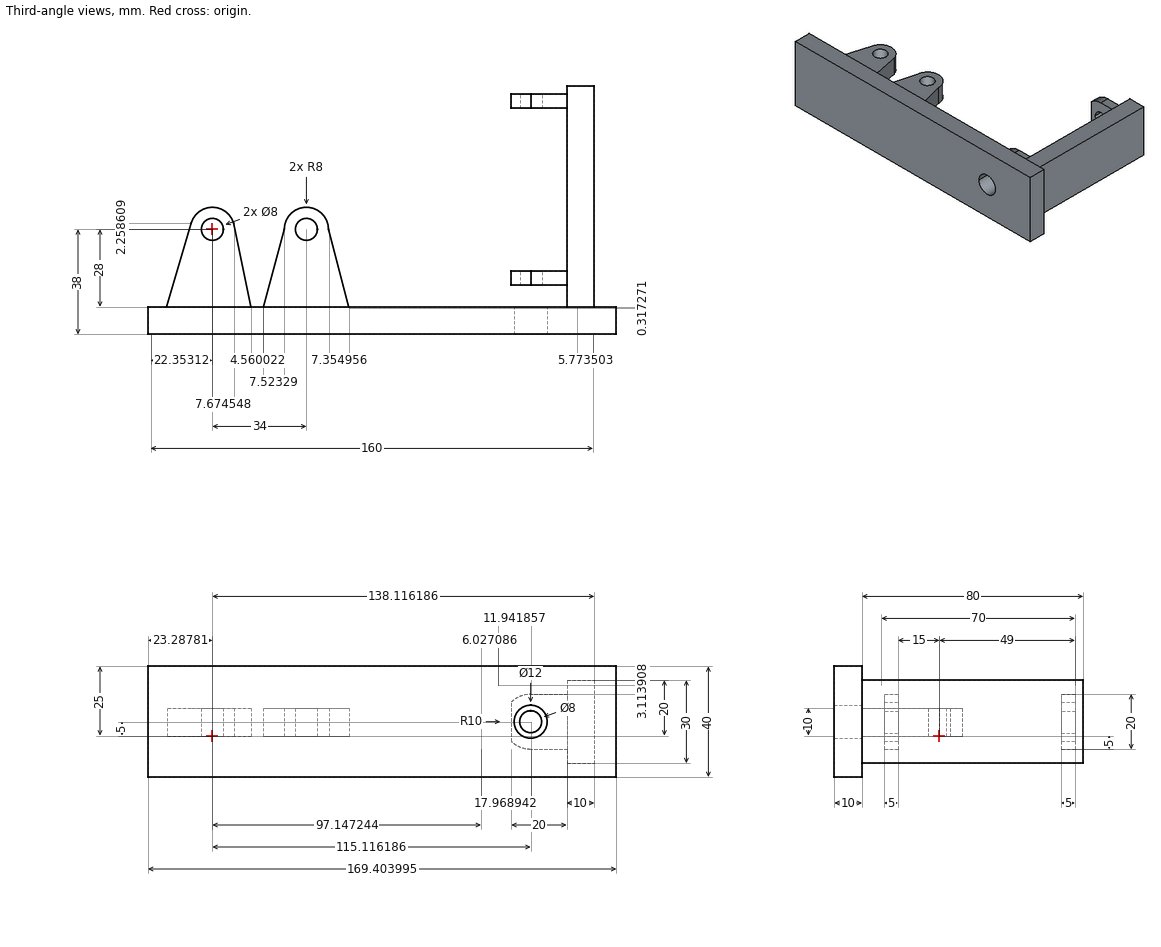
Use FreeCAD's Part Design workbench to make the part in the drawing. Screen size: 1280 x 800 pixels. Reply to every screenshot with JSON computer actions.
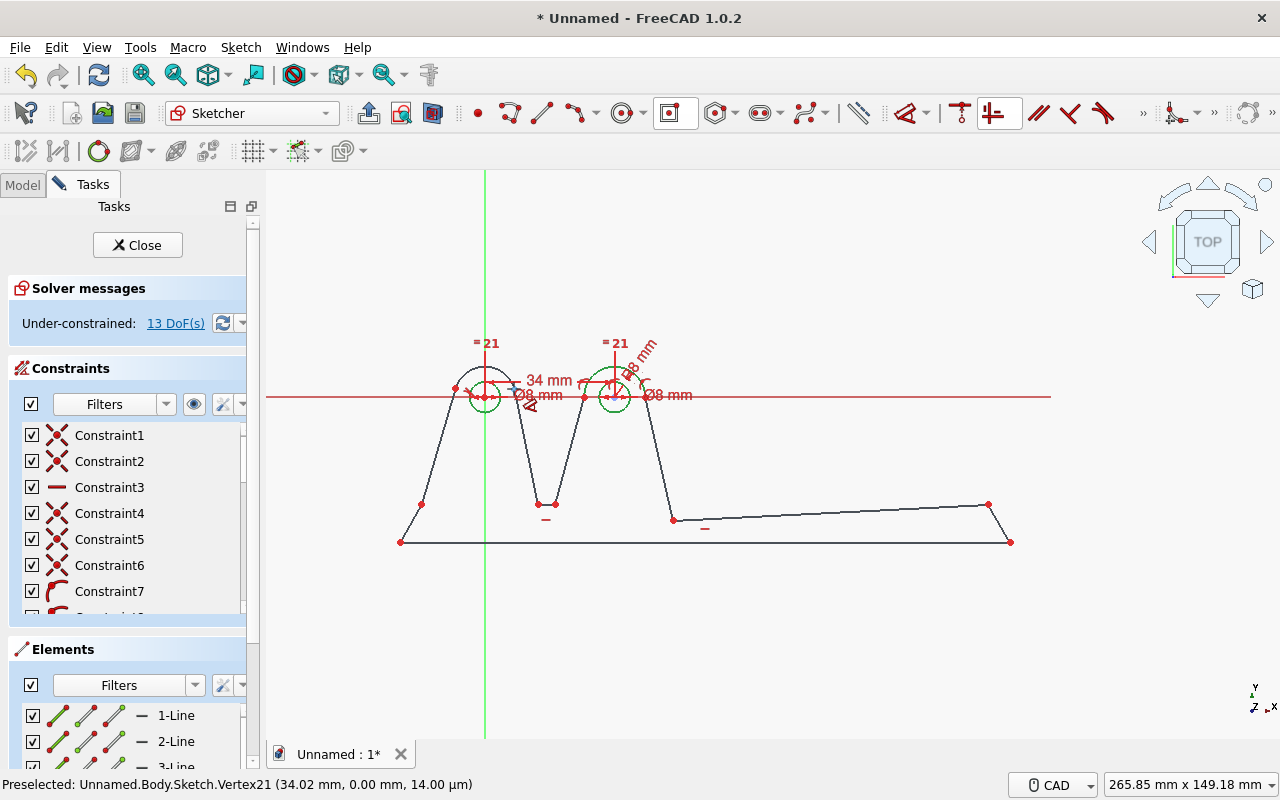
{"action": "left_click", "coordinate": [583, 543]}
{"action": "left_click", "coordinate": [705, 577]}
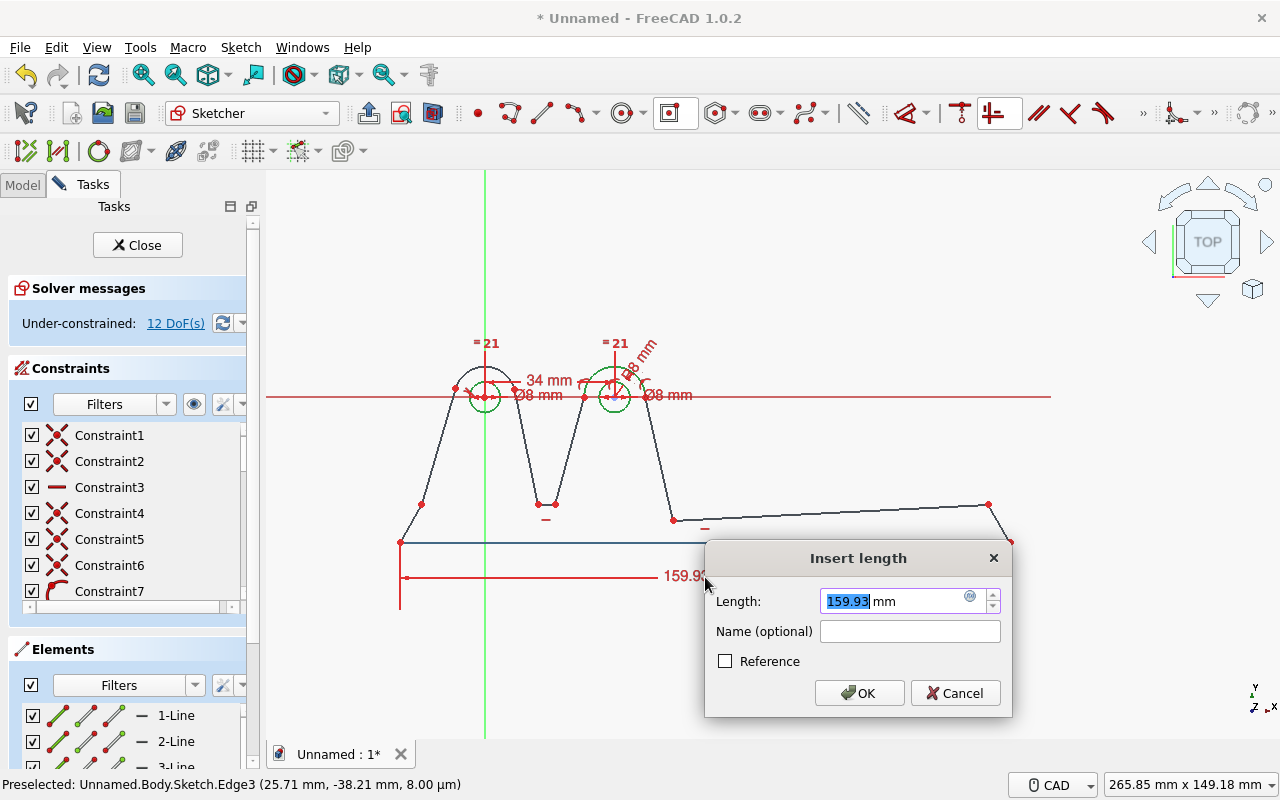
{"action": "type", "text": "160"}
{"action": "key", "text": "Return"}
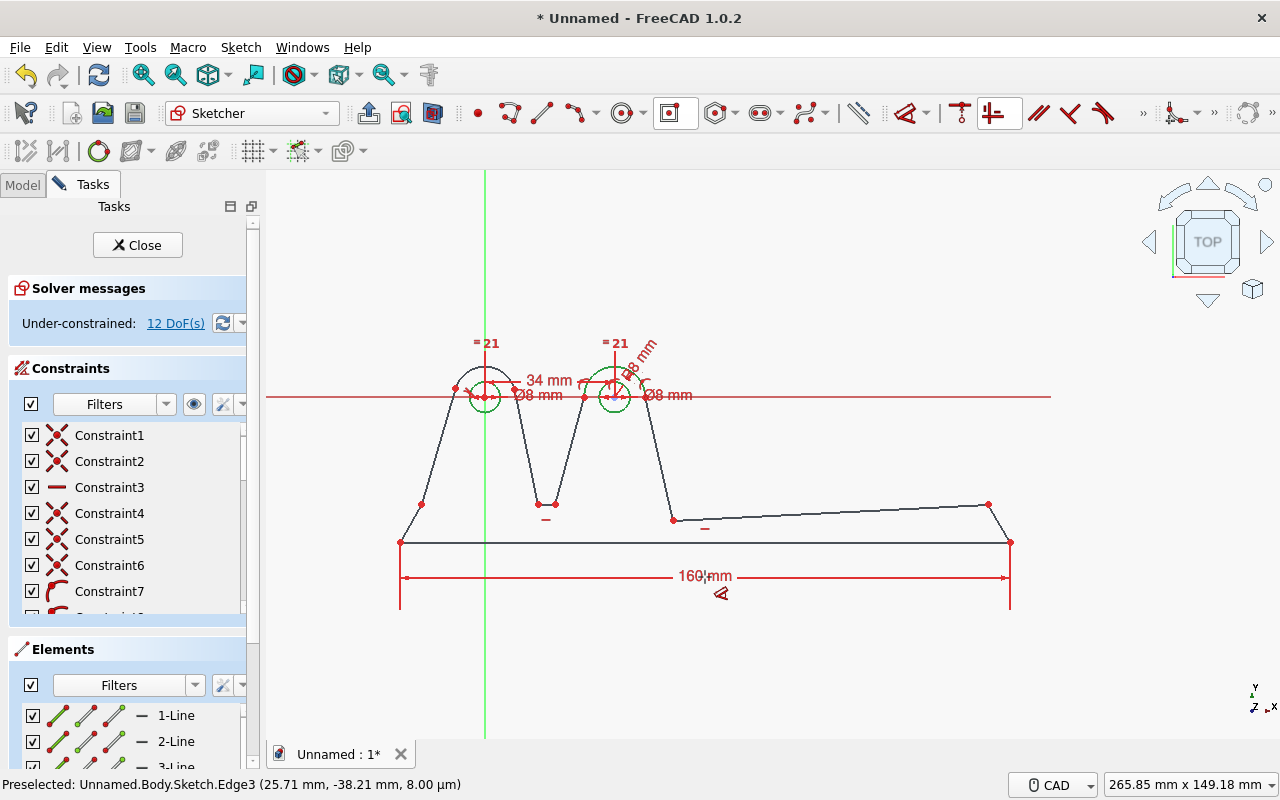
{"action": "left_click", "coordinate": [422, 505]}
{"action": "left_click", "coordinate": [388, 451]}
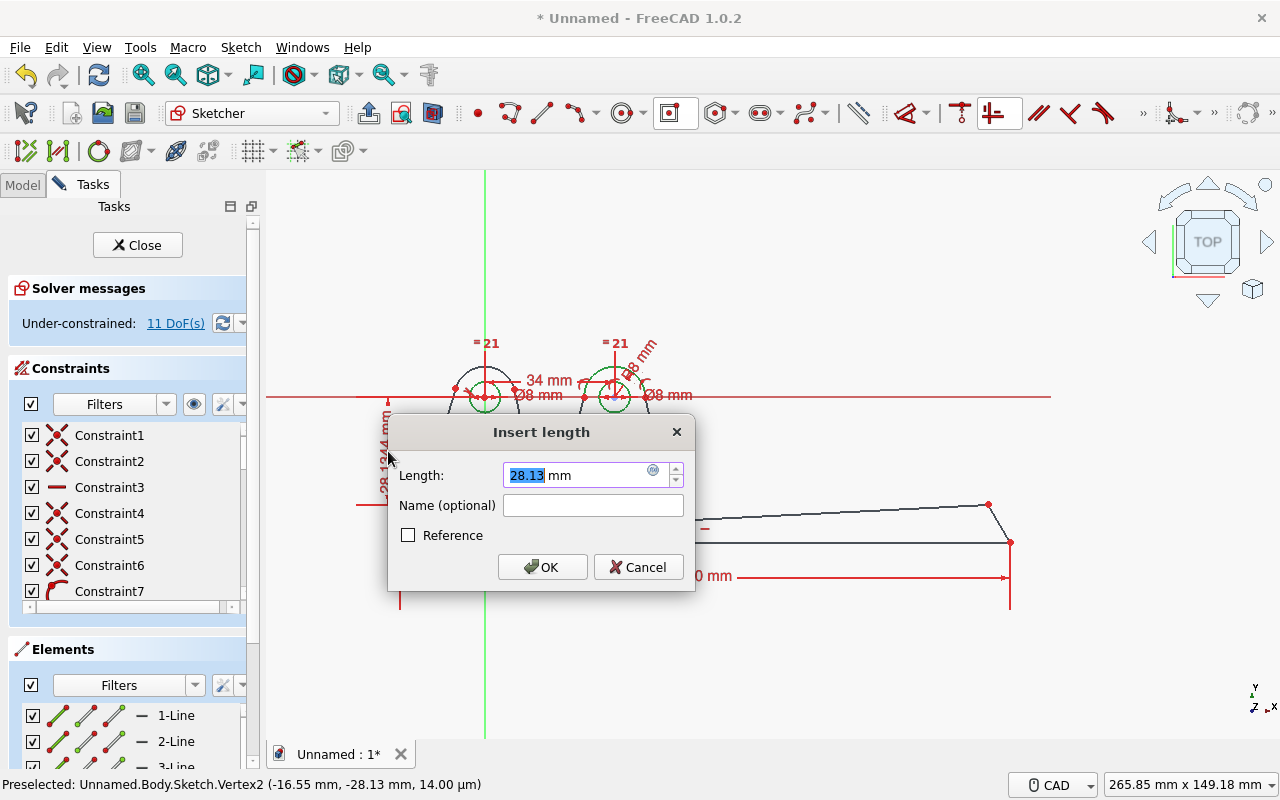
{"action": "type", "text": "28"}
{"action": "key", "text": "Return"}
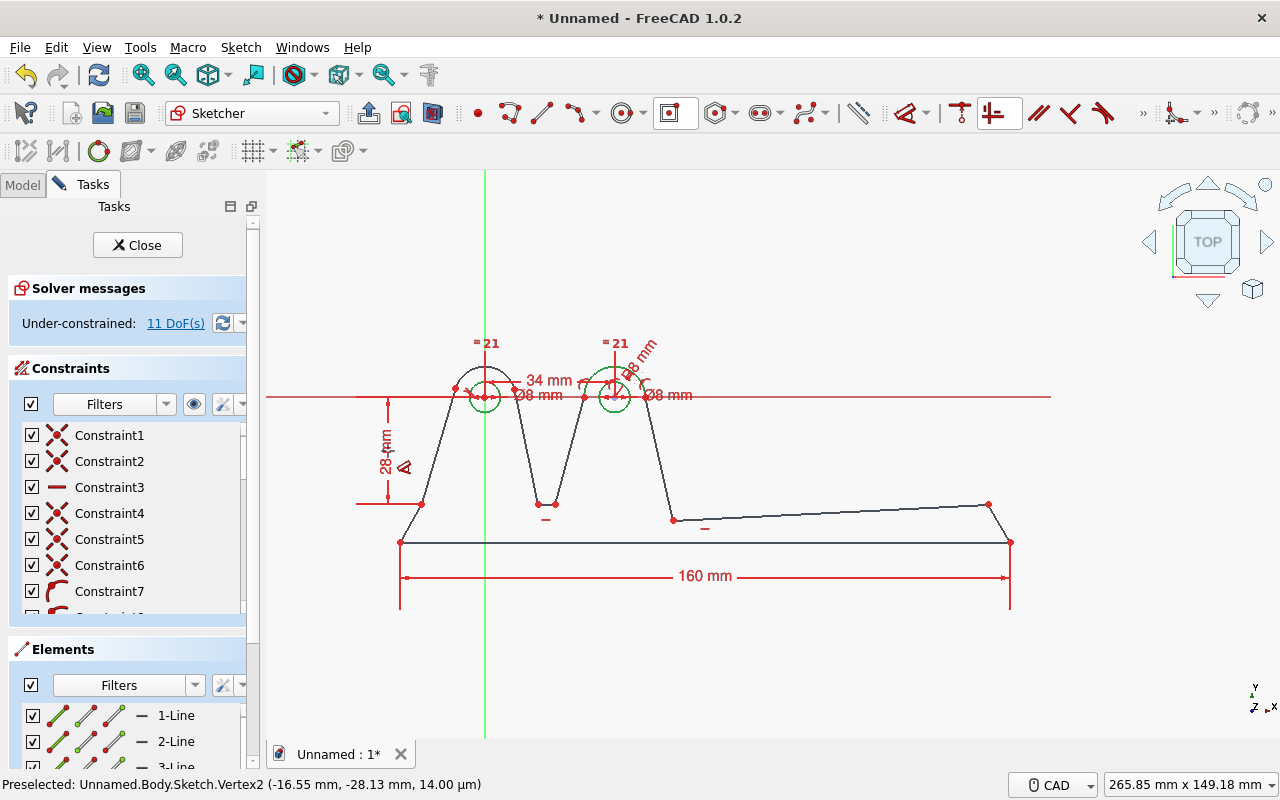
{"action": "left_click", "coordinate": [400, 543]}
{"action": "left_click", "coordinate": [366, 504]}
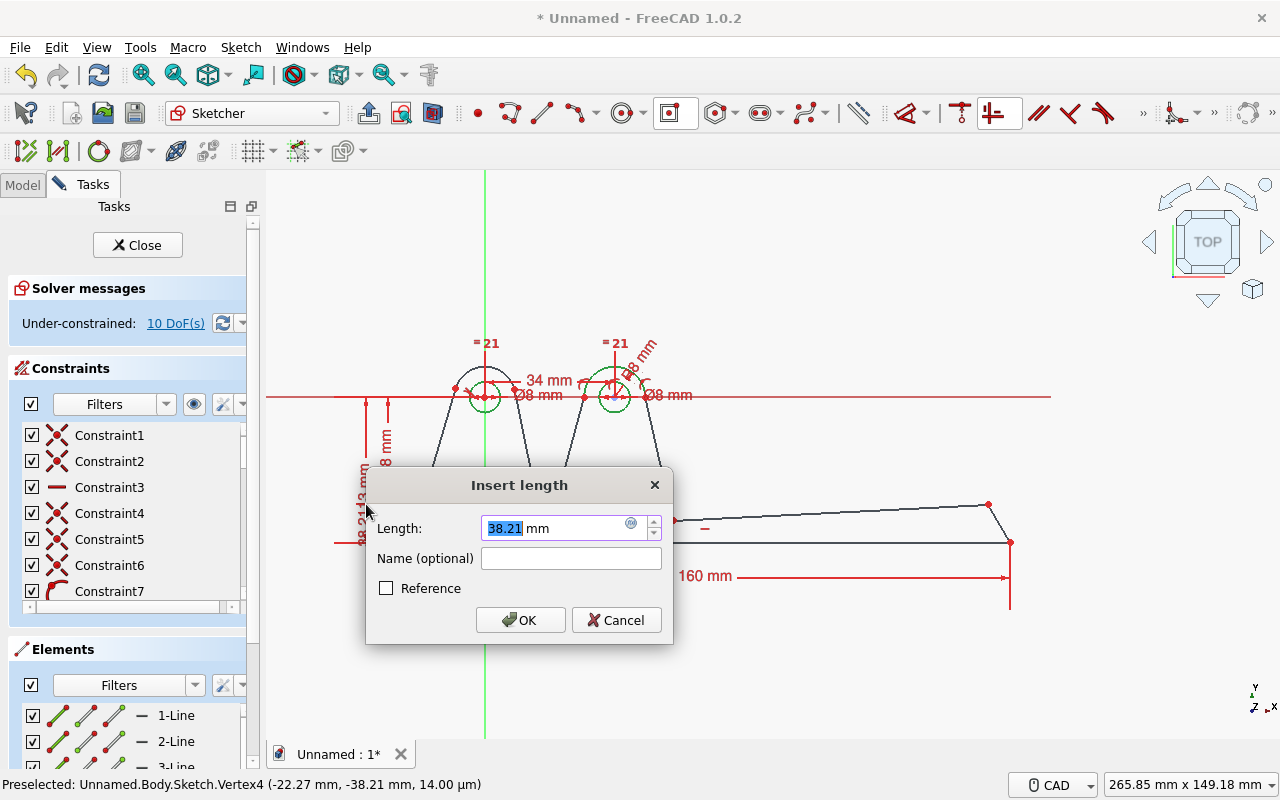
{"action": "type", "text": "38"}
{"action": "key", "text": "Return"}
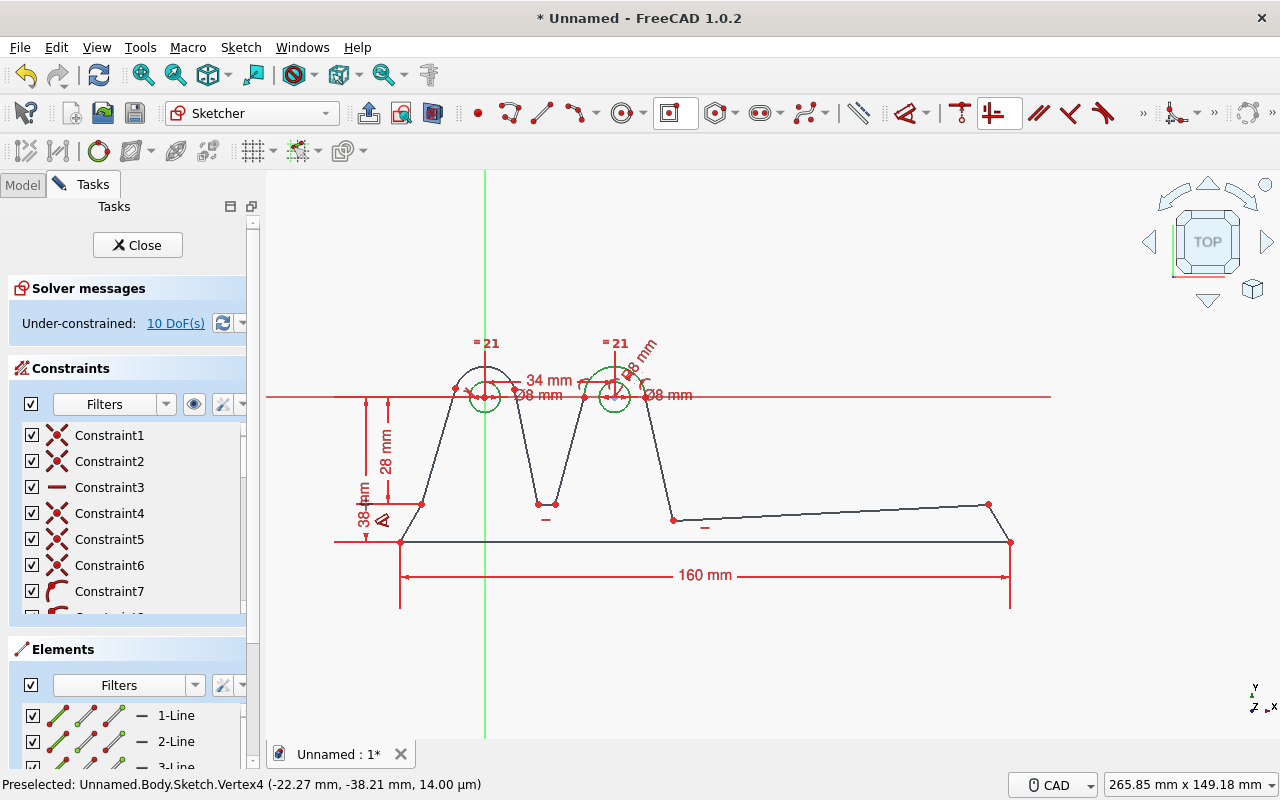
{"action": "left_click", "coordinate": [988, 505]}
{"action": "left_click", "coordinate": [1022, 451]}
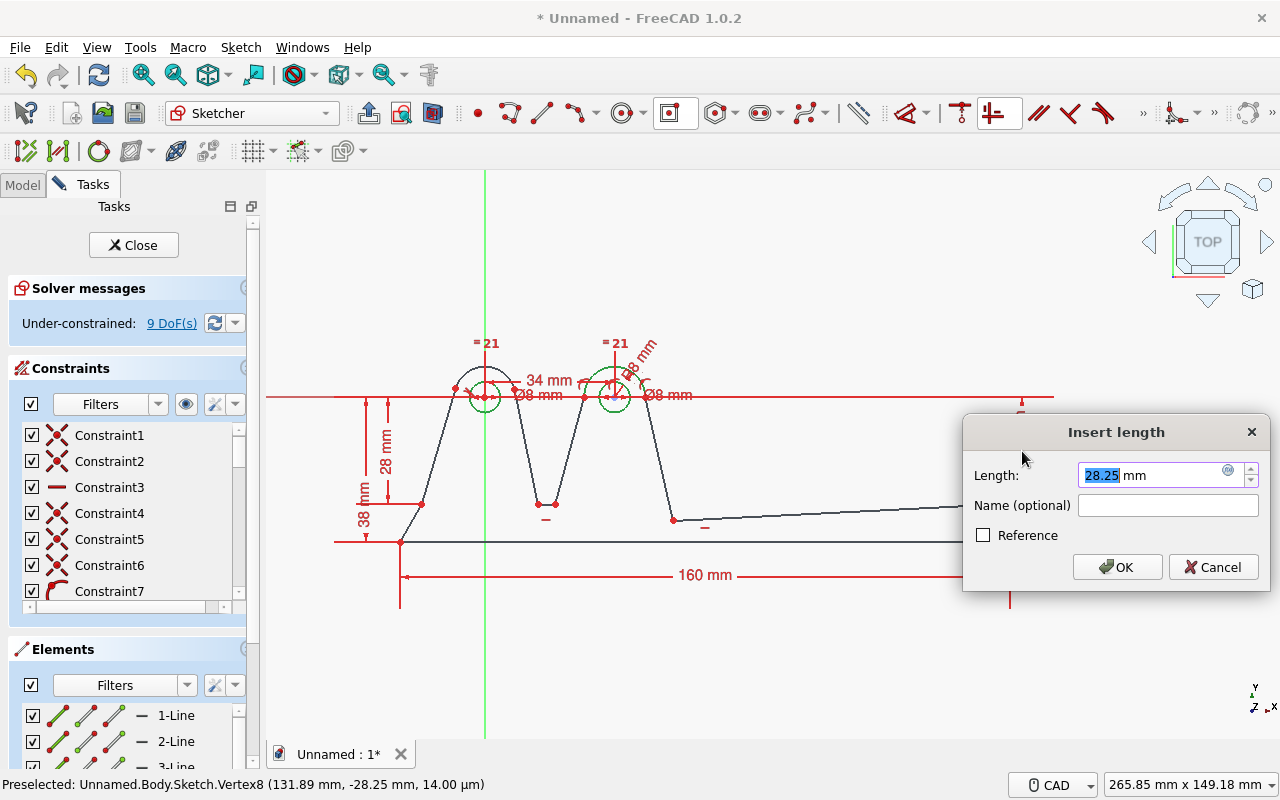
{"action": "type", "text": "28"}
{"action": "key", "text": "Return"}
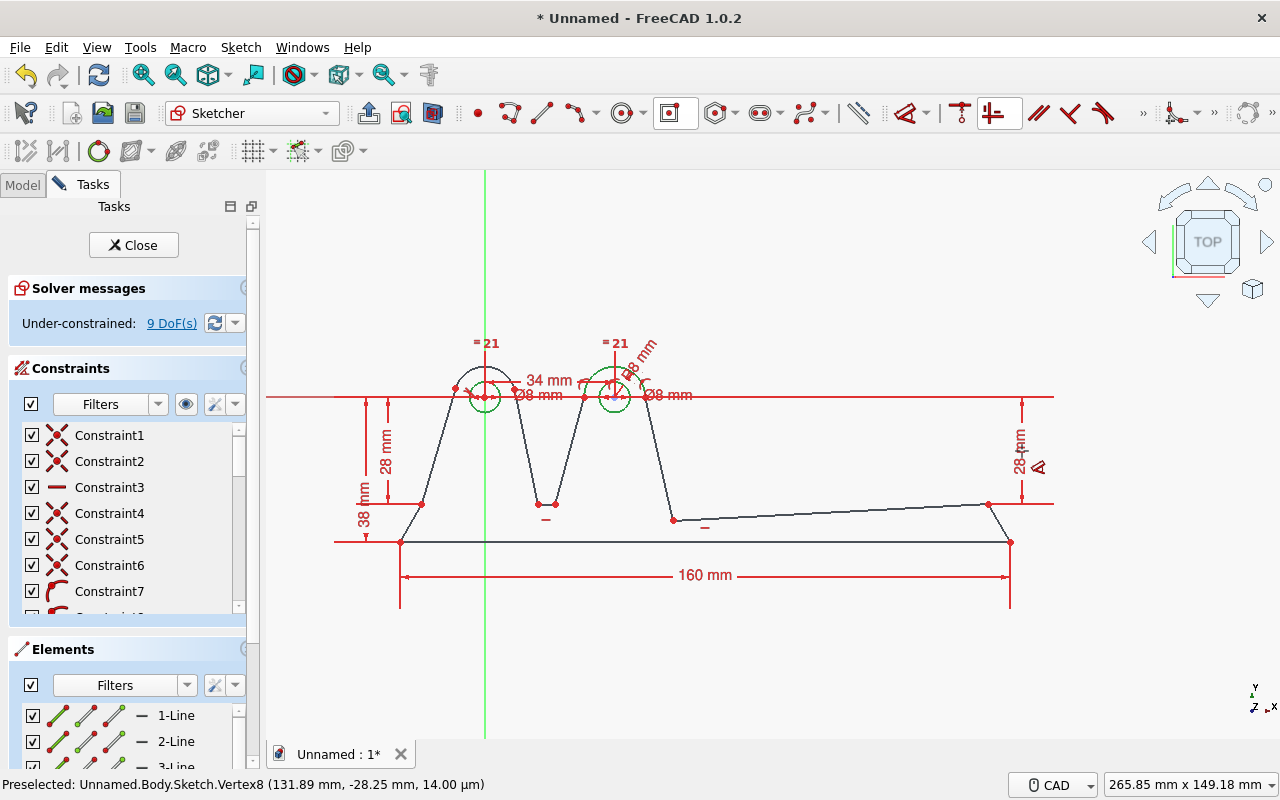
{"action": "left_click", "coordinate": [555, 505]}
{"action": "left_click", "coordinate": [451, 476]}